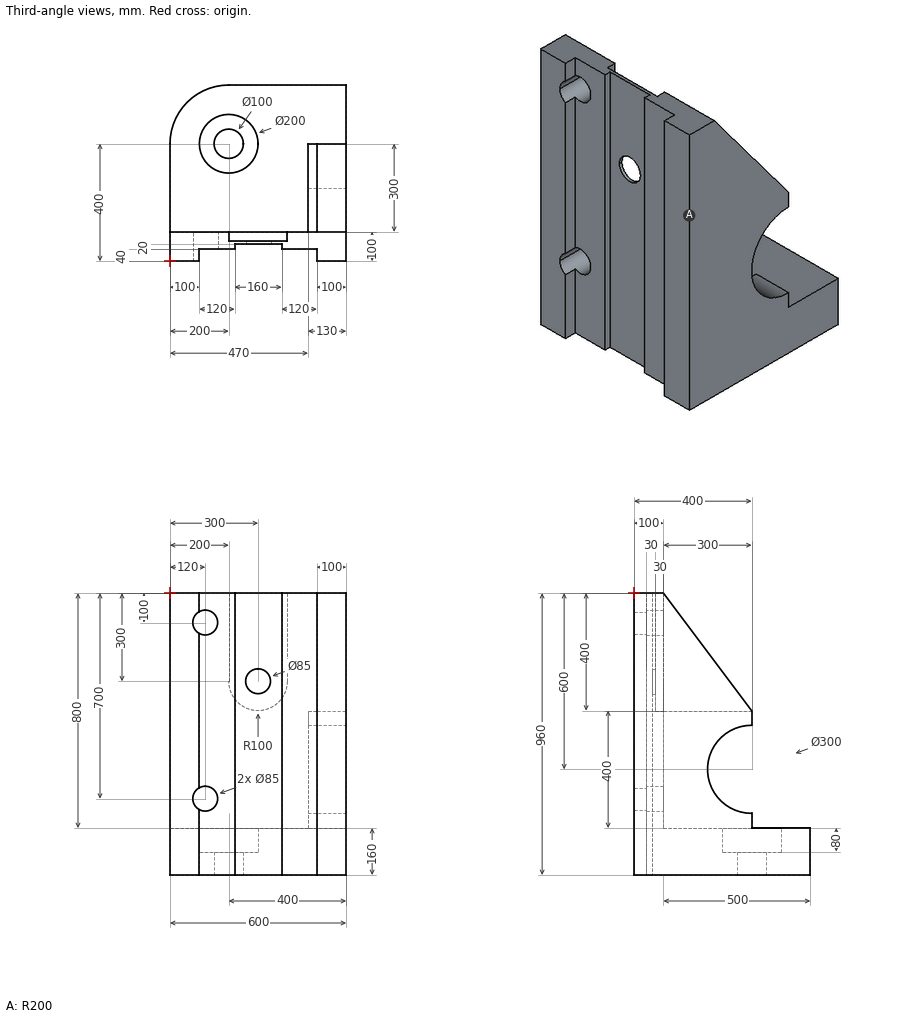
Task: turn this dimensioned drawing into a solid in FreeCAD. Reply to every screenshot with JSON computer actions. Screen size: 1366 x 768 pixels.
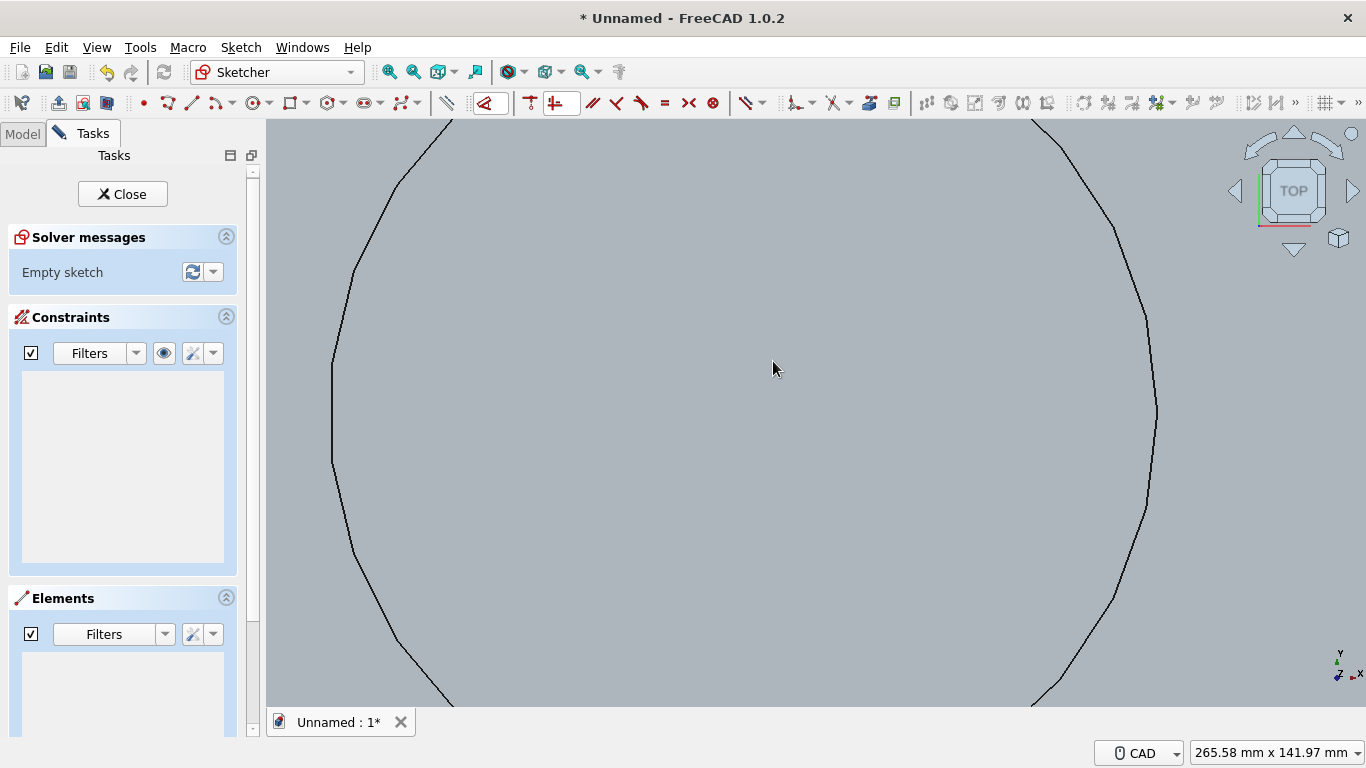
{"action": "left_click", "coordinate": [254, 104]}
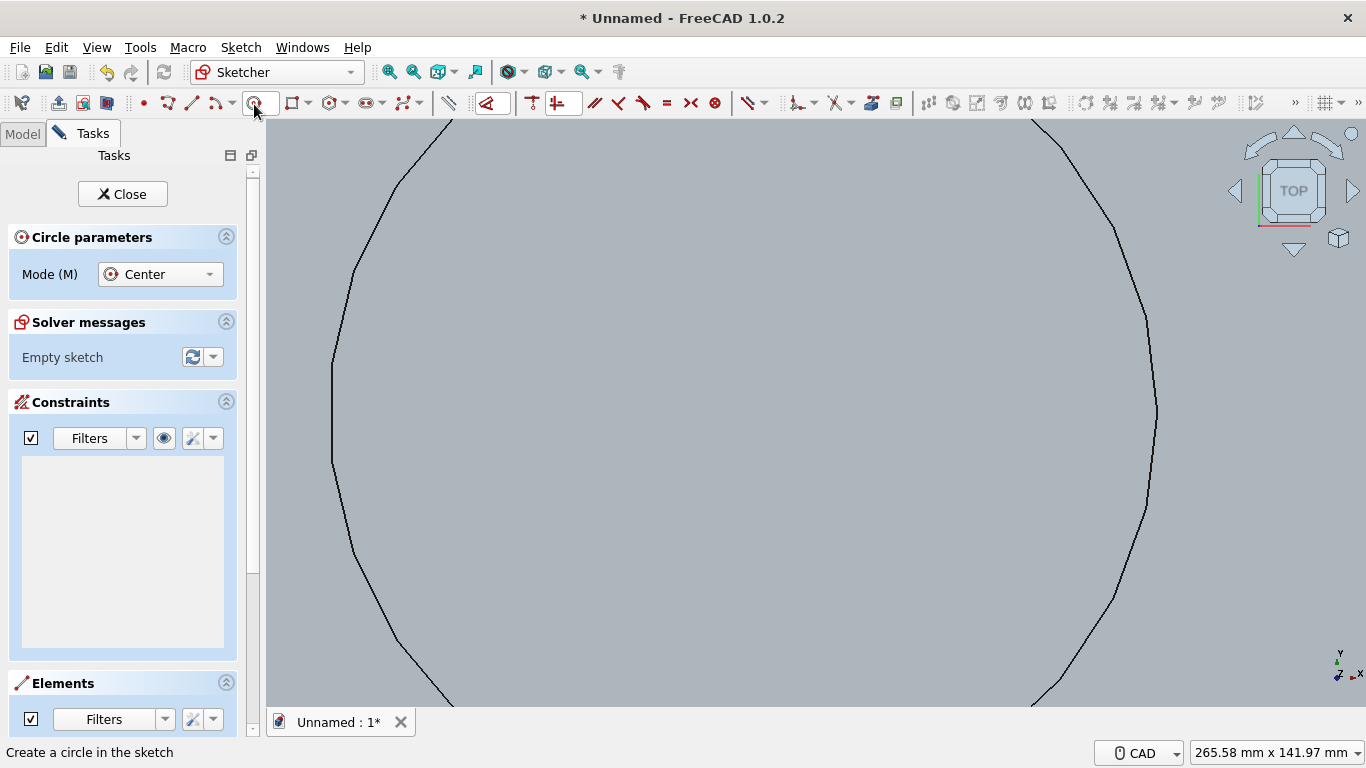
{"action": "left_click", "coordinate": [743, 413]}
{"action": "left_click", "coordinate": [890, 266]}
{"action": "key", "text": "Escape"}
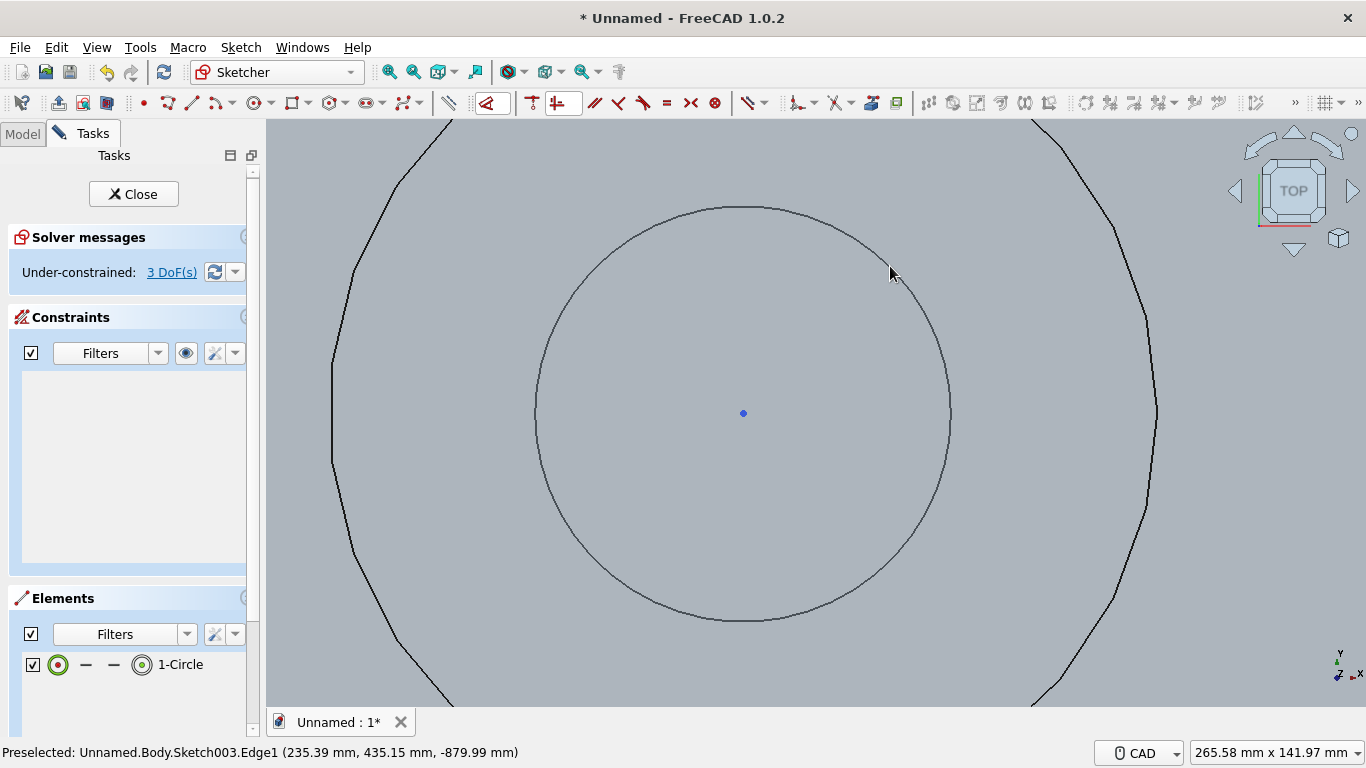
{"action": "left_click", "coordinate": [890, 267]}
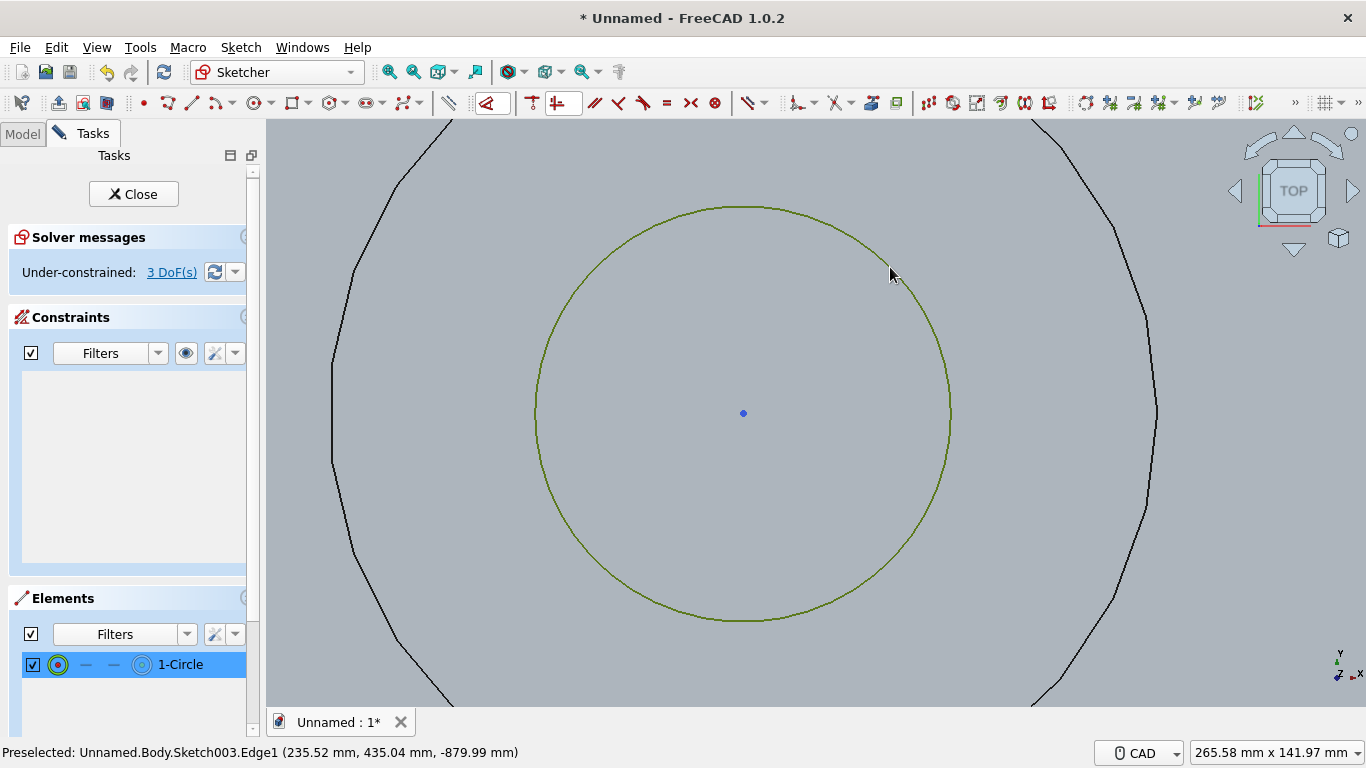
{"action": "key", "text": "k o"}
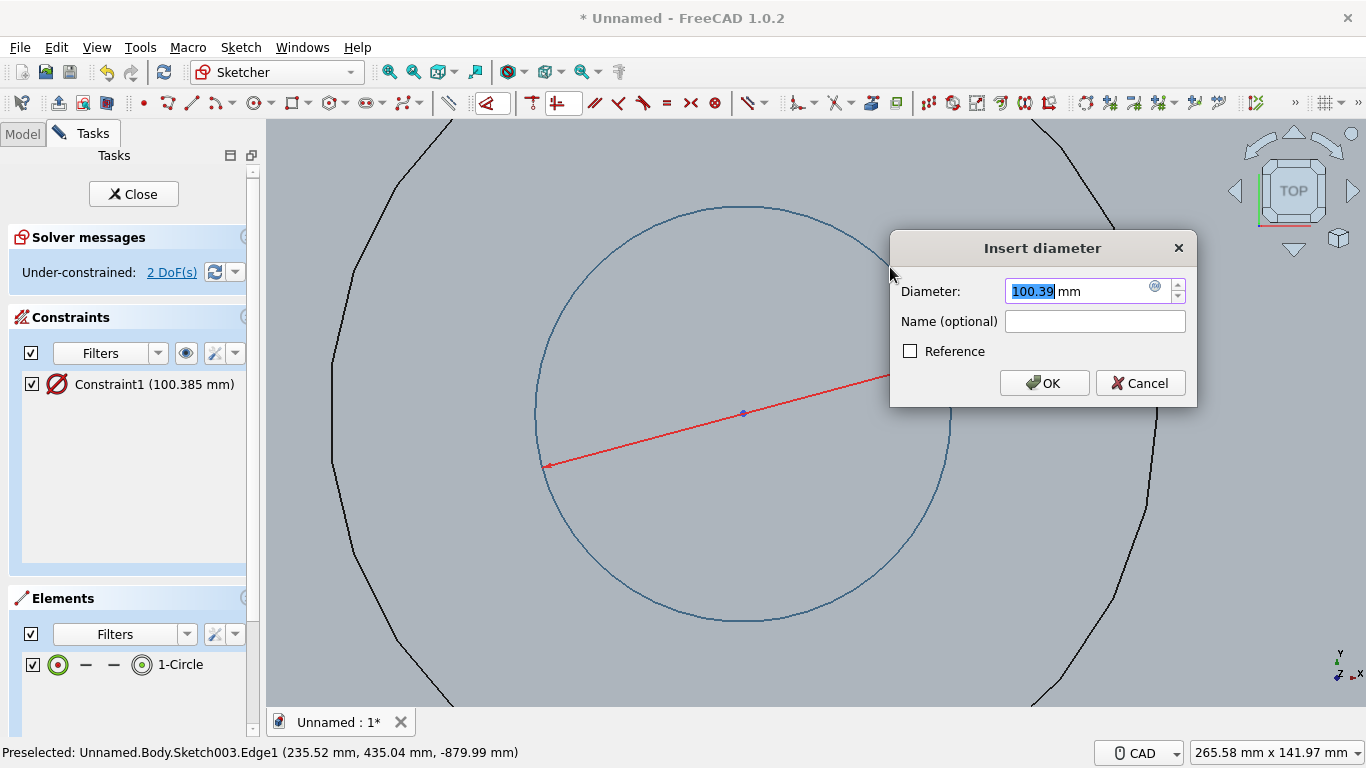
{"action": "type", "text": "100"}
{"action": "key", "text": "Return"}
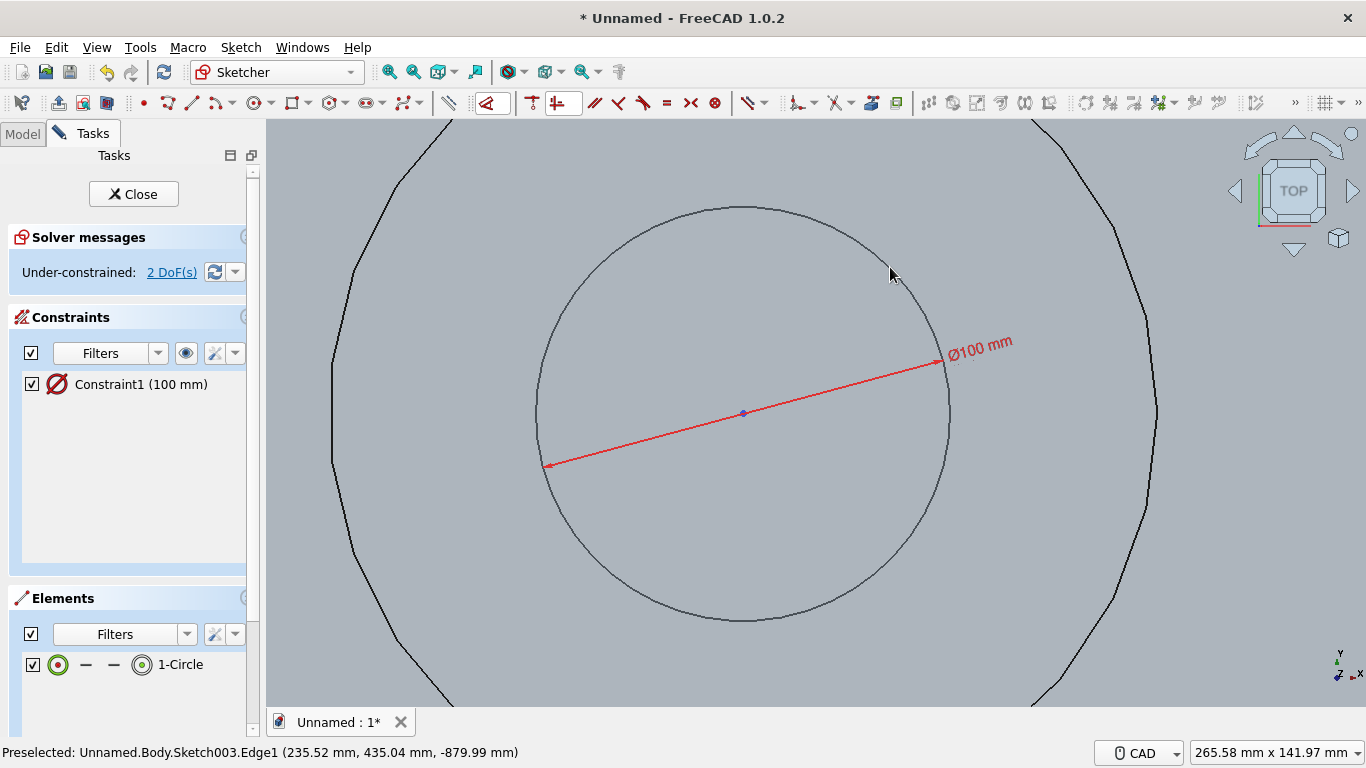
{"action": "left_click", "coordinate": [743, 414]}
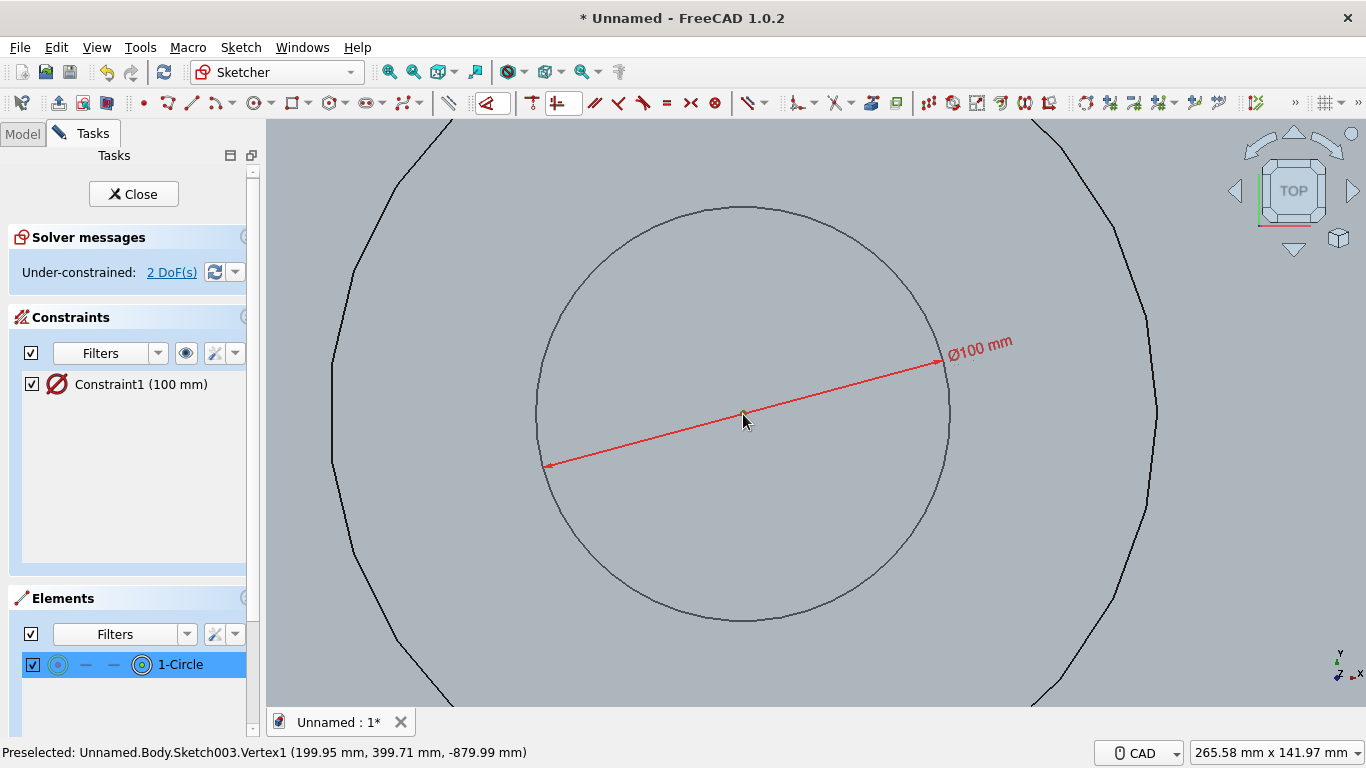
{"action": "key", "text": "l"}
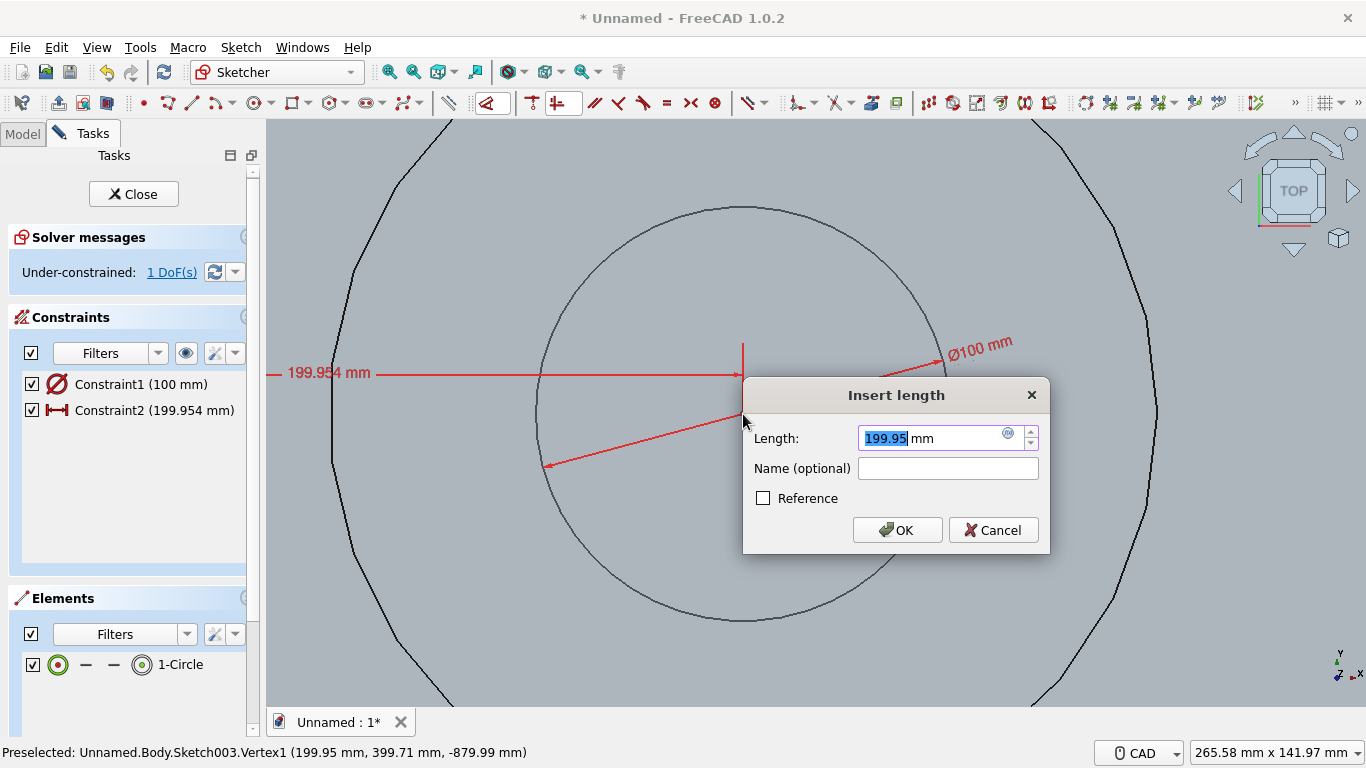
{"action": "type", "text": "200"}
{"action": "key", "text": "Return"}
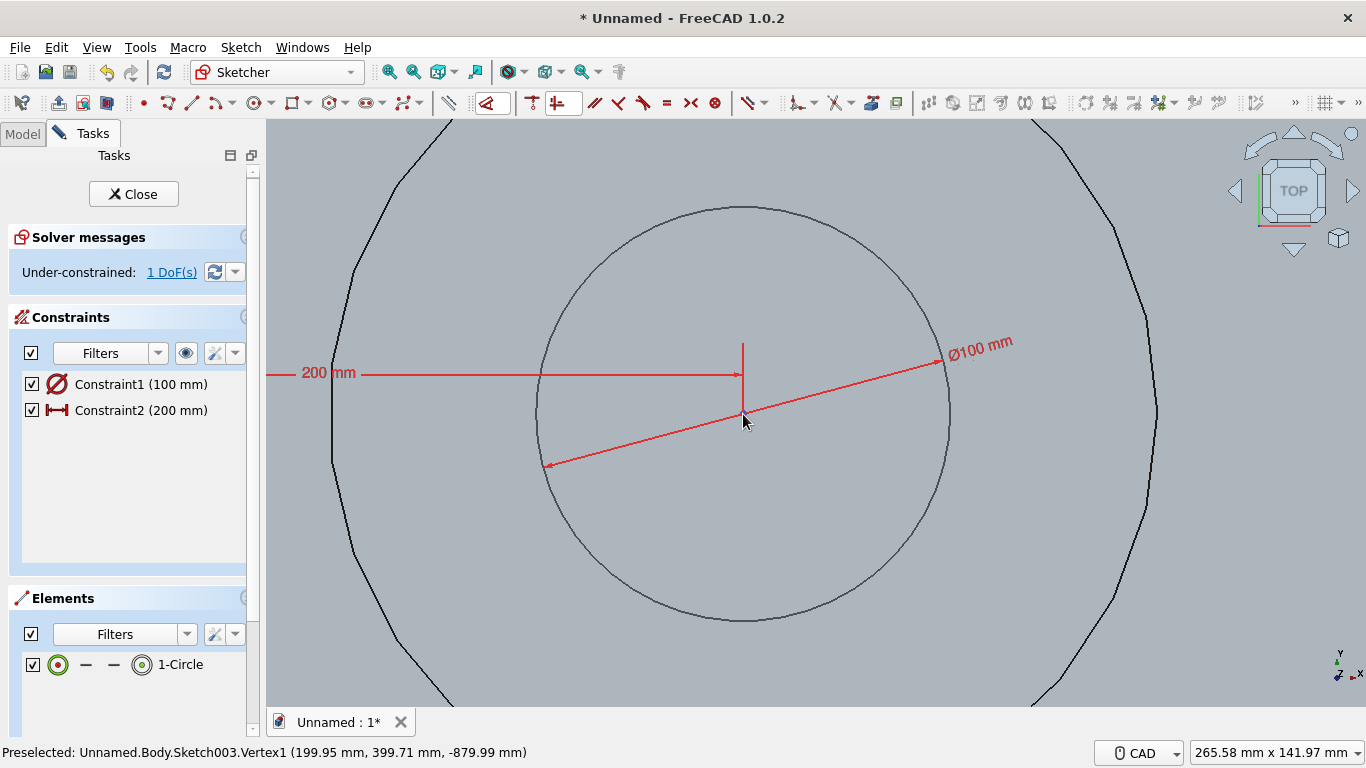
{"action": "left_click", "coordinate": [743, 414]}